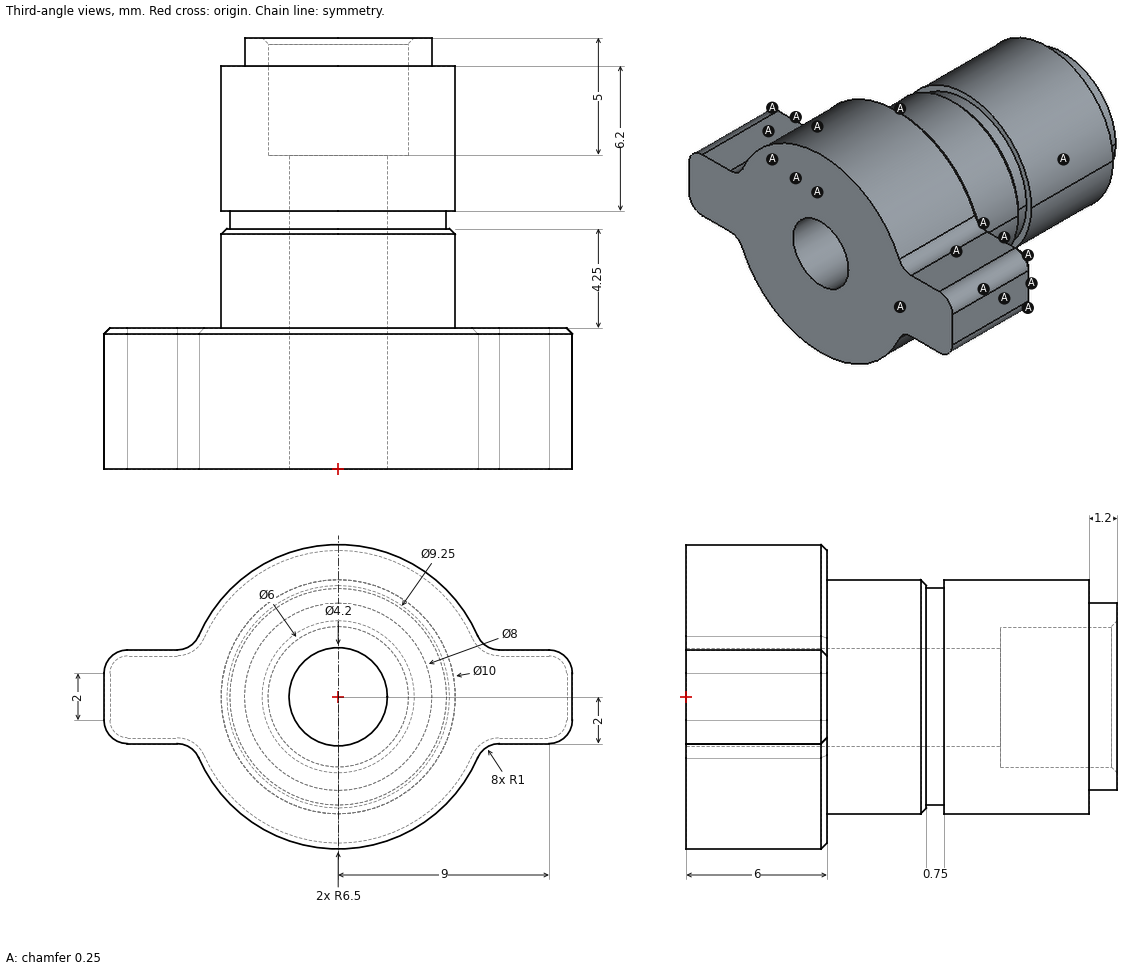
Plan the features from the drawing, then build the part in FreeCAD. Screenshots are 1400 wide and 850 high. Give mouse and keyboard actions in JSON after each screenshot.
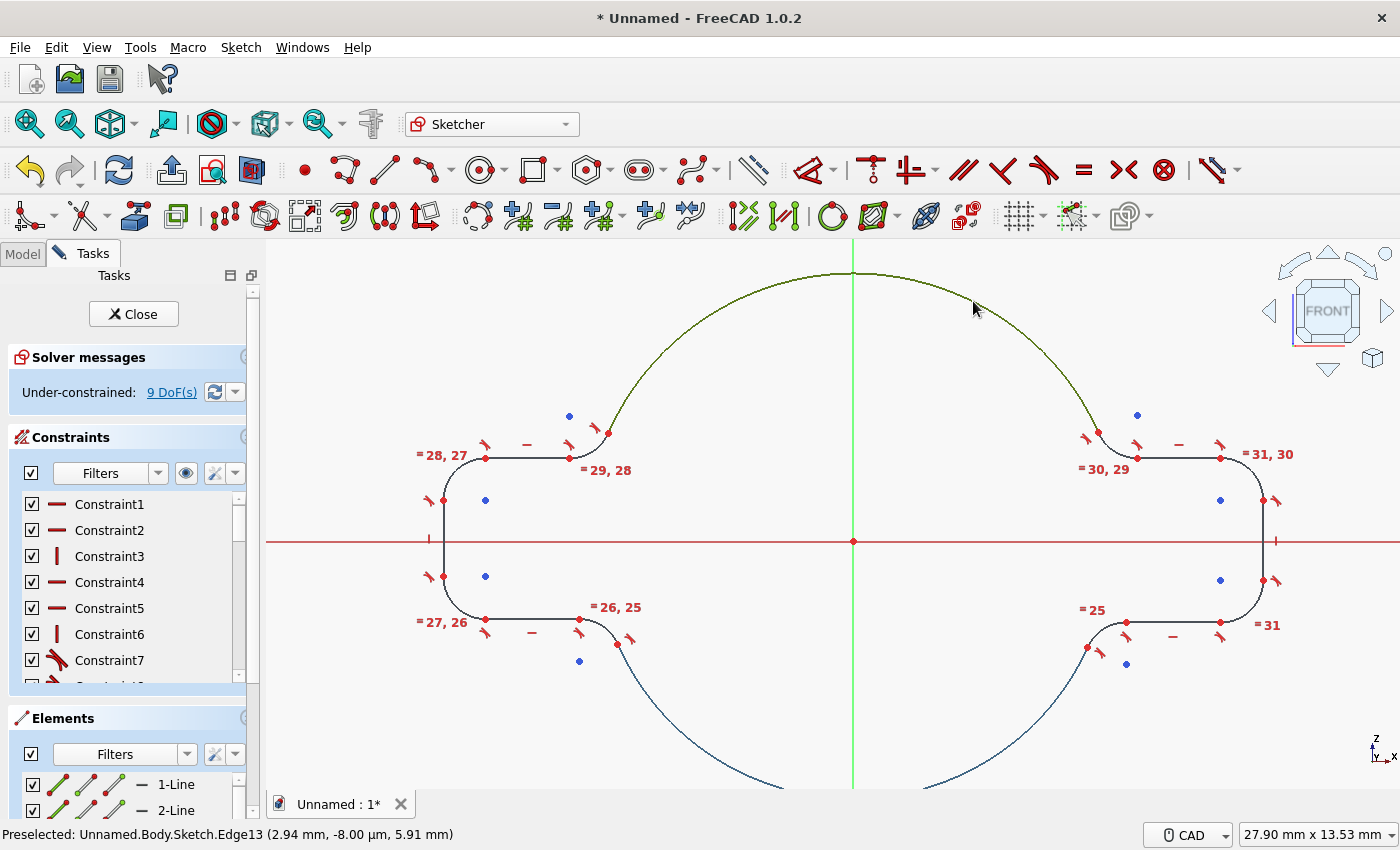
{"action": "left_click", "coordinate": [1084, 170]}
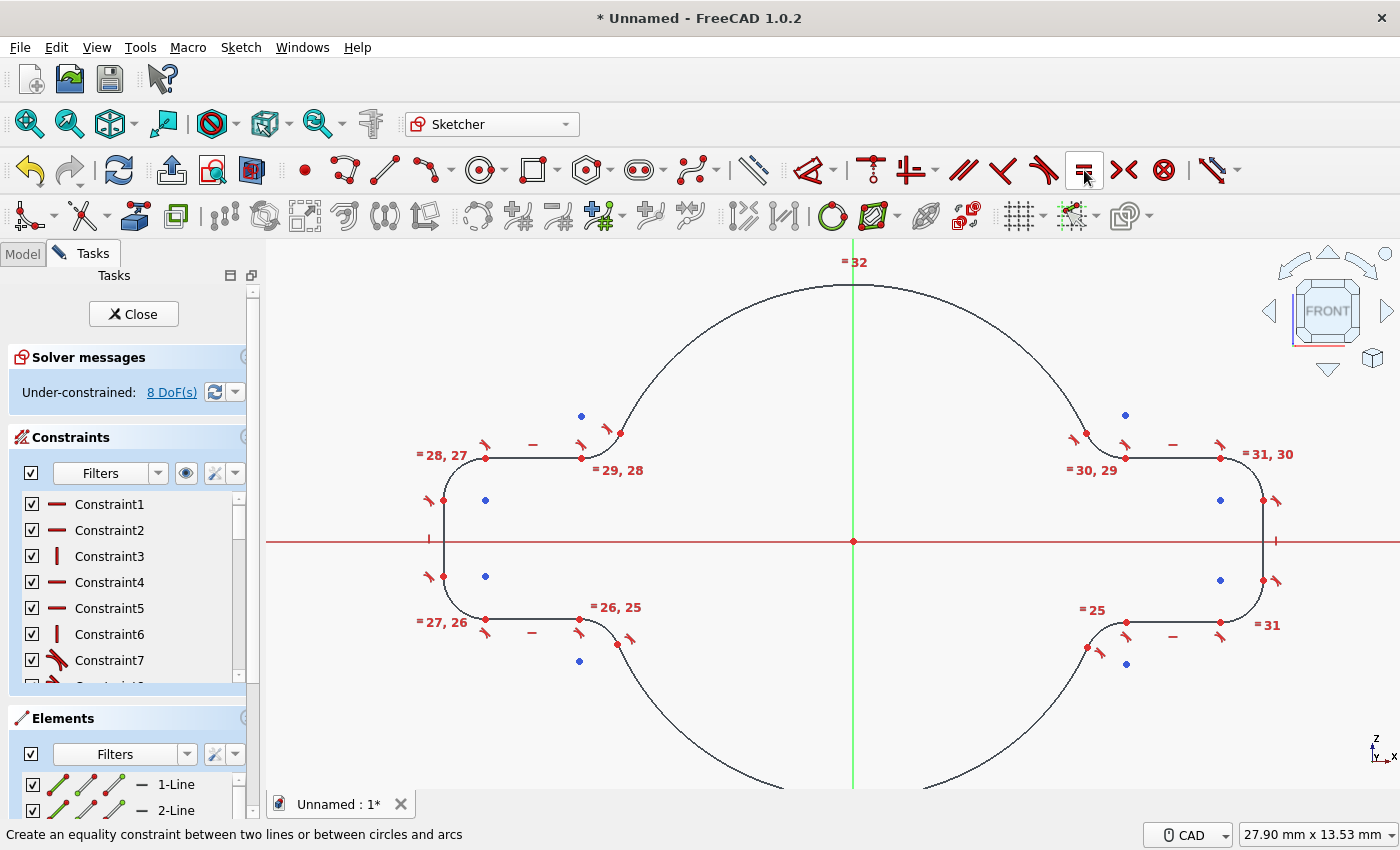
{"action": "left_click", "coordinate": [486, 501]}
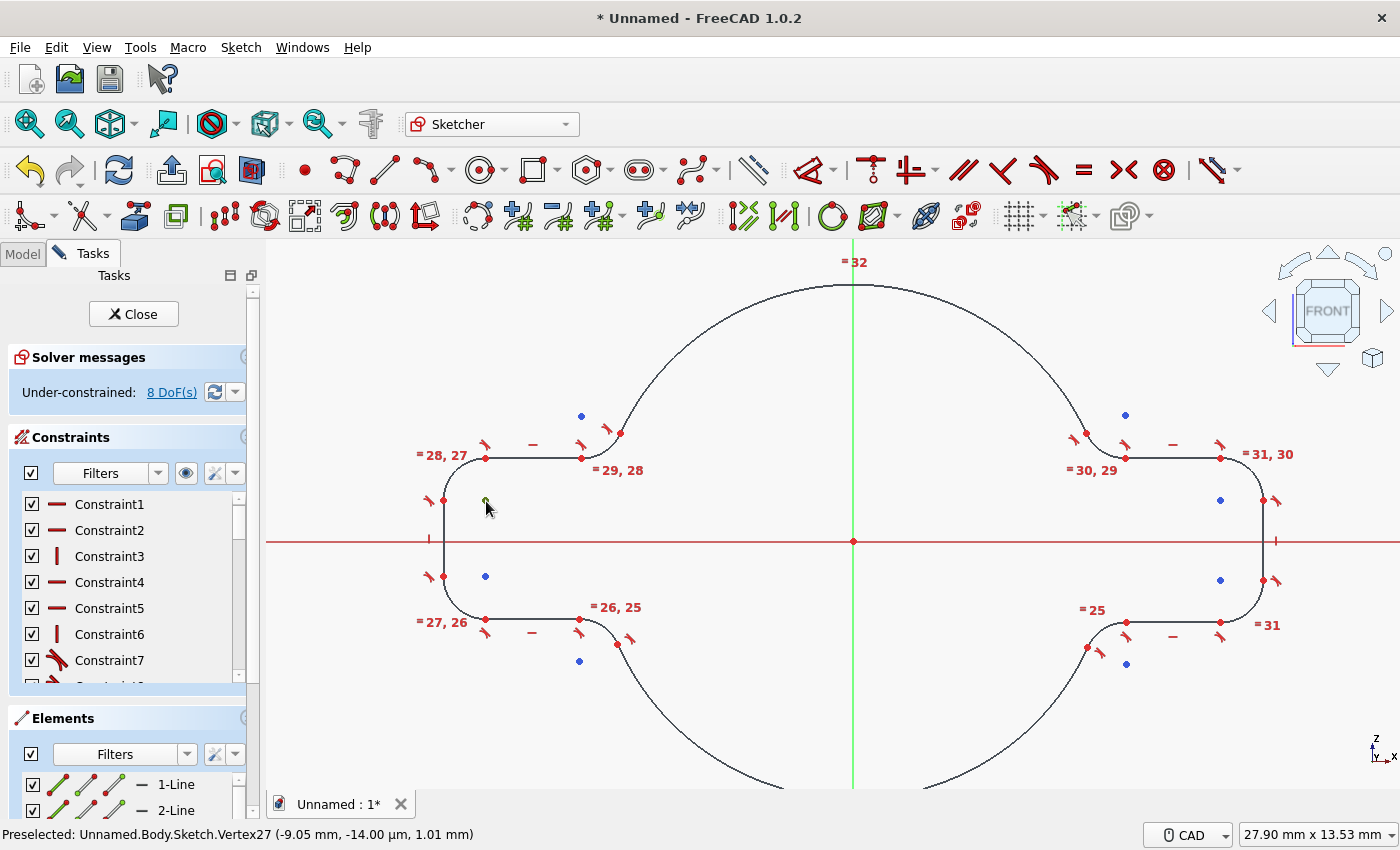
{"action": "left_click", "coordinate": [1221, 500]}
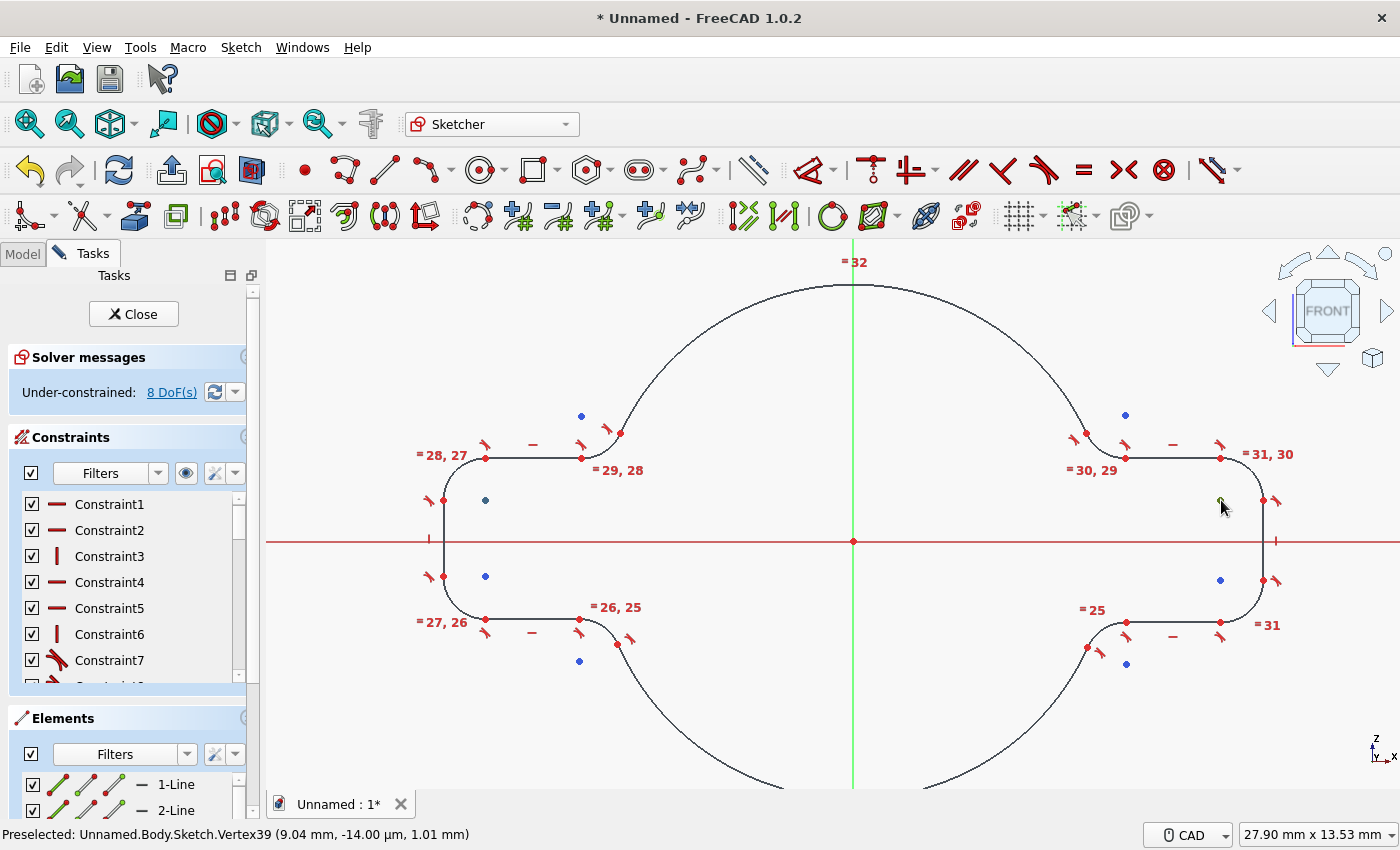
{"action": "left_click", "coordinate": [853, 726]}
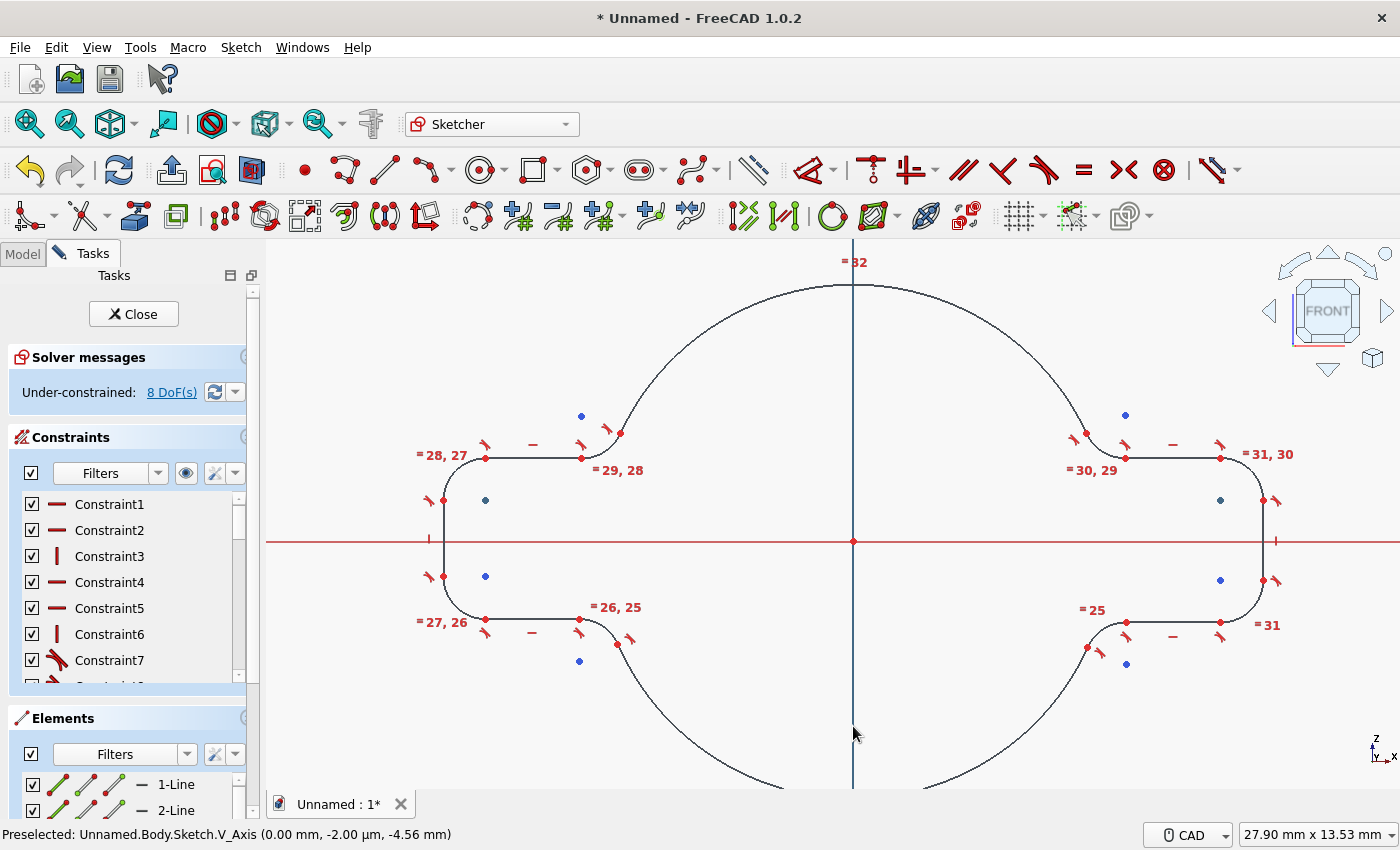
{"action": "left_click", "coordinate": [1124, 170]}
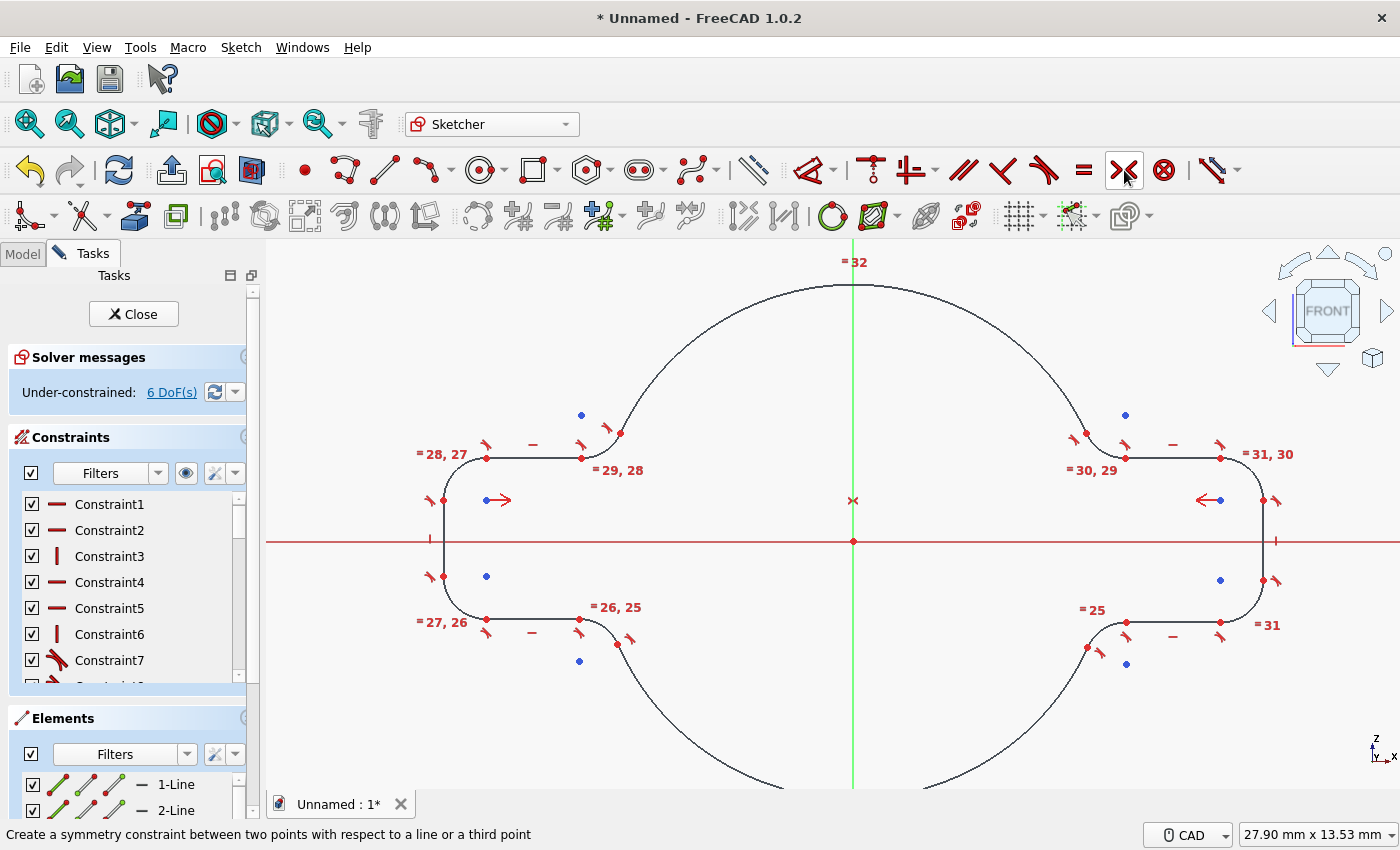
{"action": "left_click", "coordinate": [1112, 625]}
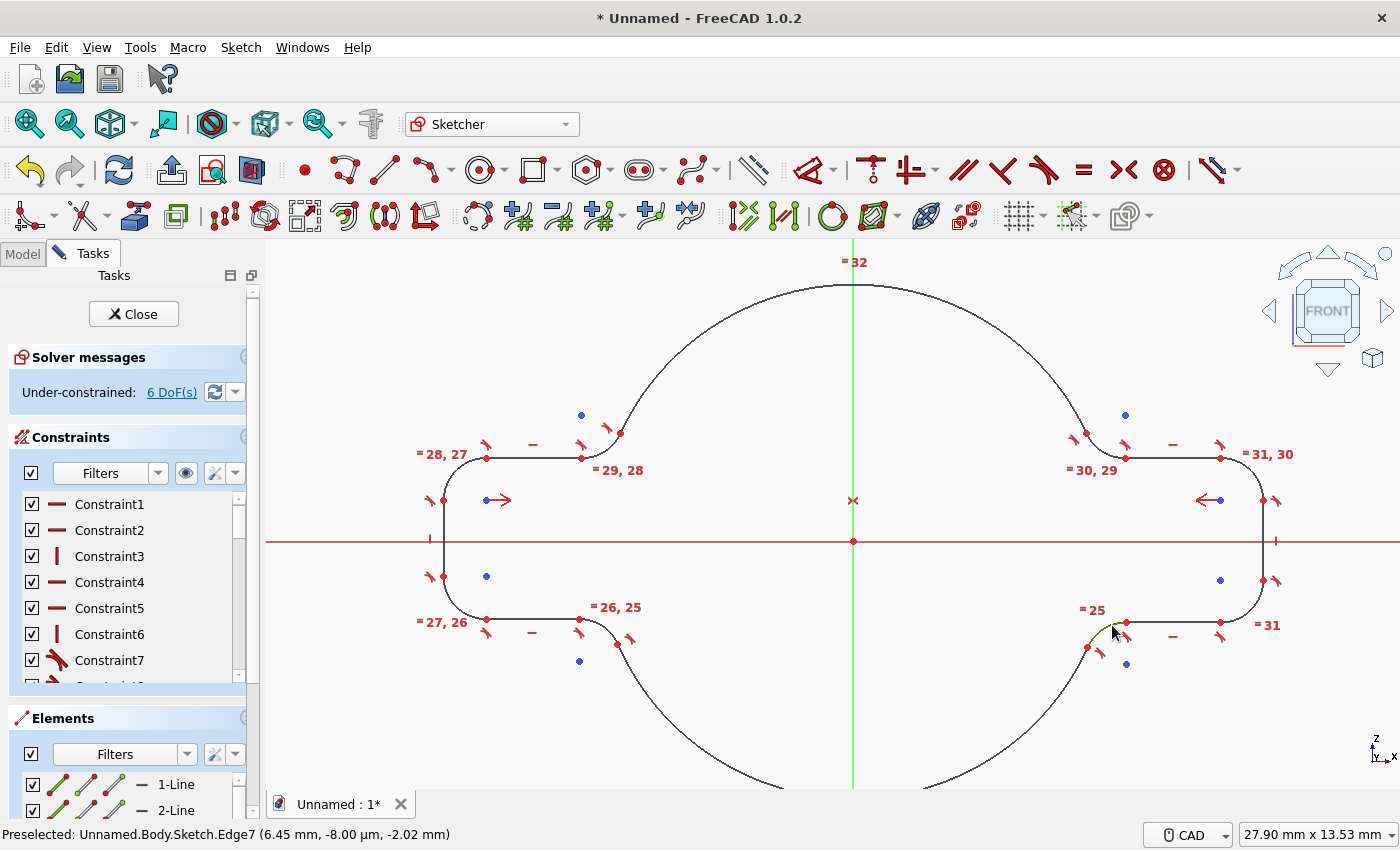
{"action": "left_click", "coordinate": [836, 170]}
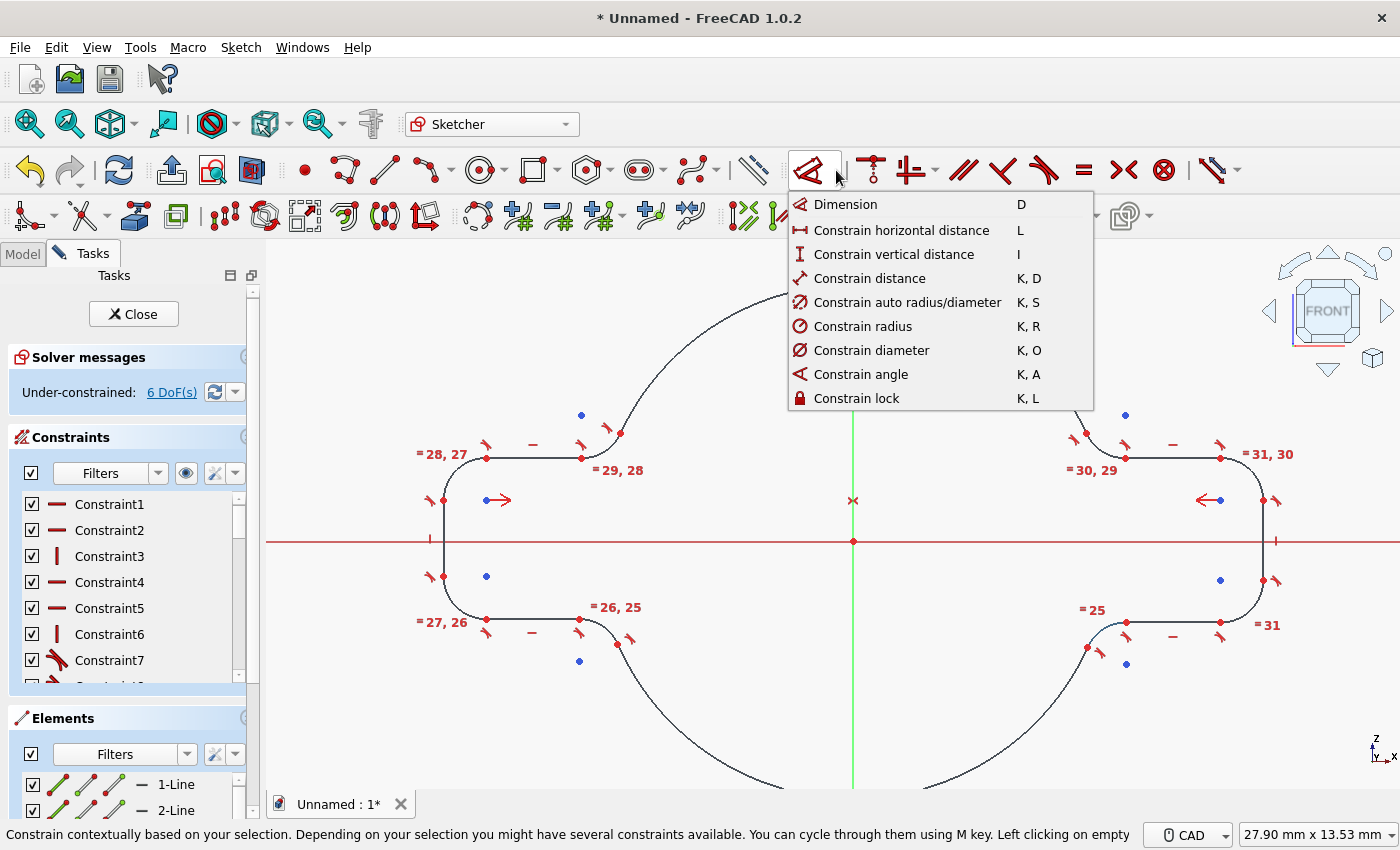
{"action": "left_click", "coordinate": [941, 326]}